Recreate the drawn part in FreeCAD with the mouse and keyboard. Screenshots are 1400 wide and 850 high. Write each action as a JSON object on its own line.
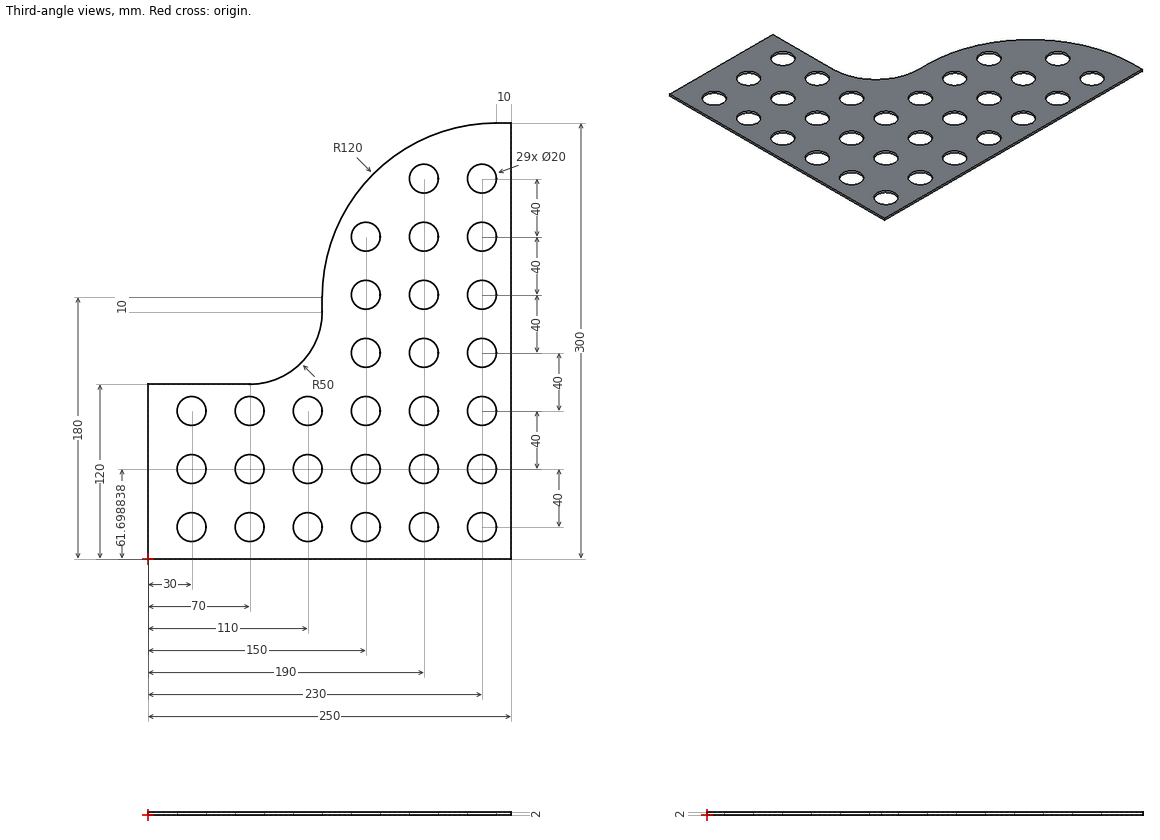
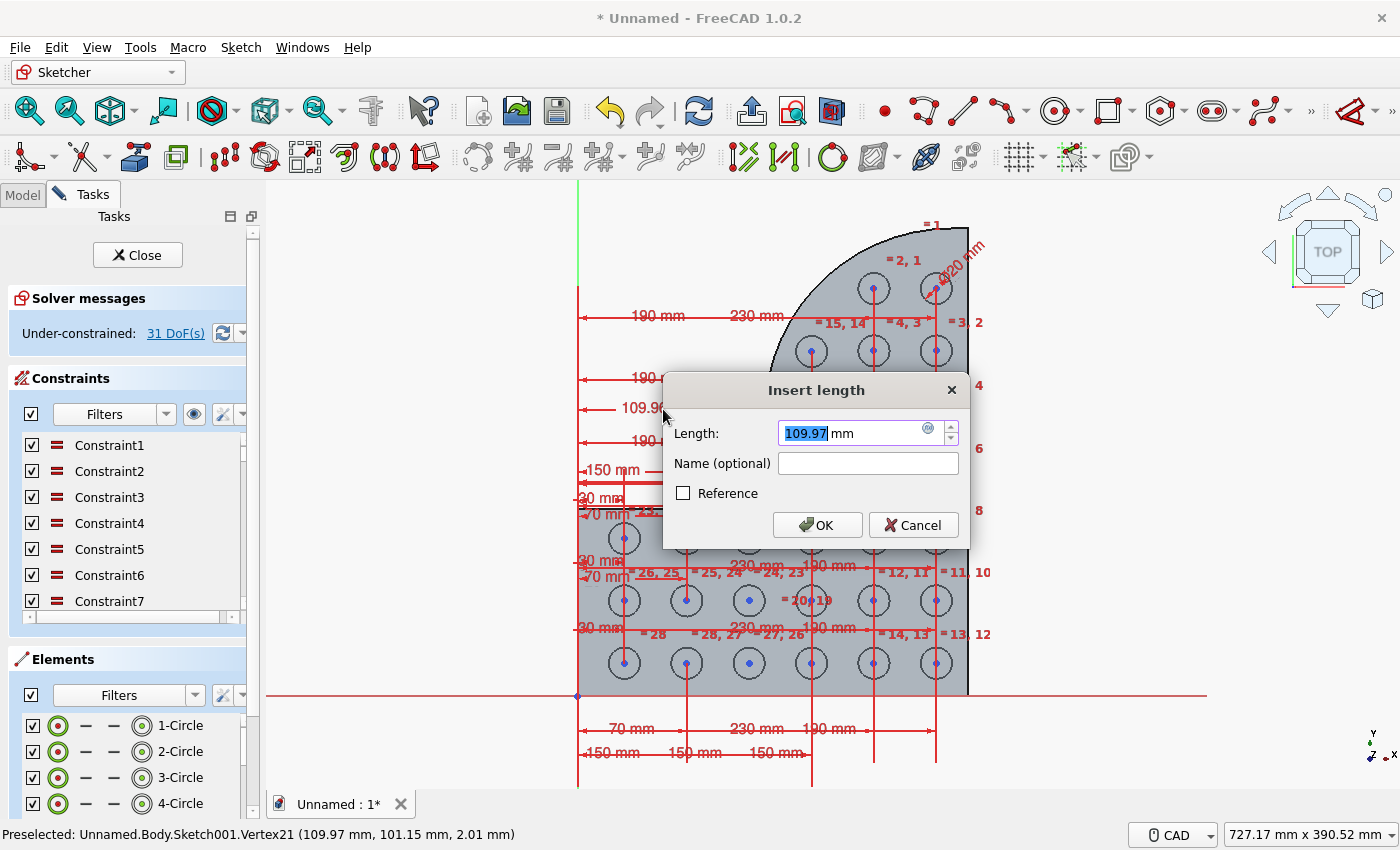
{"action": "type", "text": "110"}
{"action": "key", "text": "Return"}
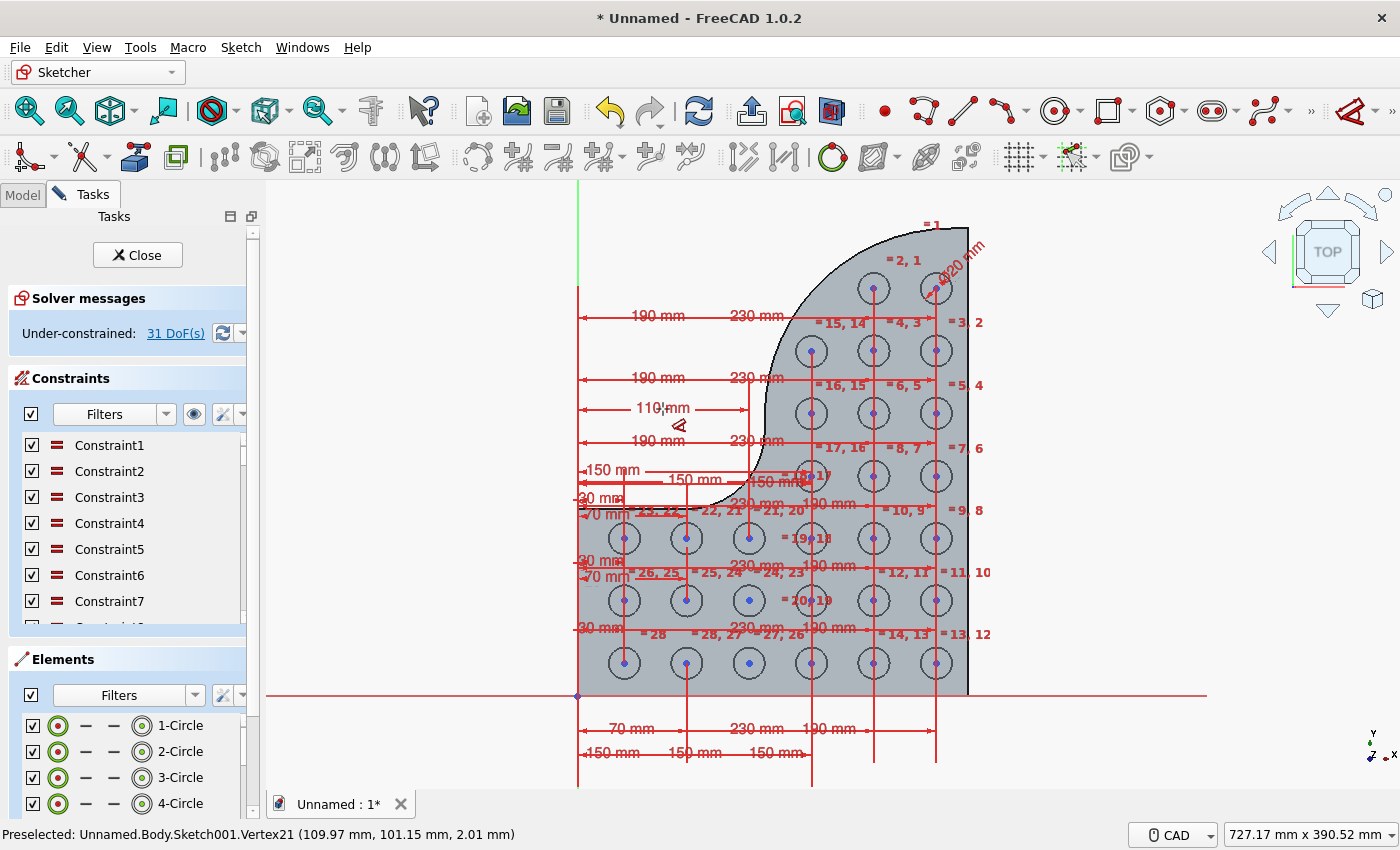
{"action": "left_click", "coordinate": [749, 601]}
{"action": "left_click", "coordinate": [703, 730]}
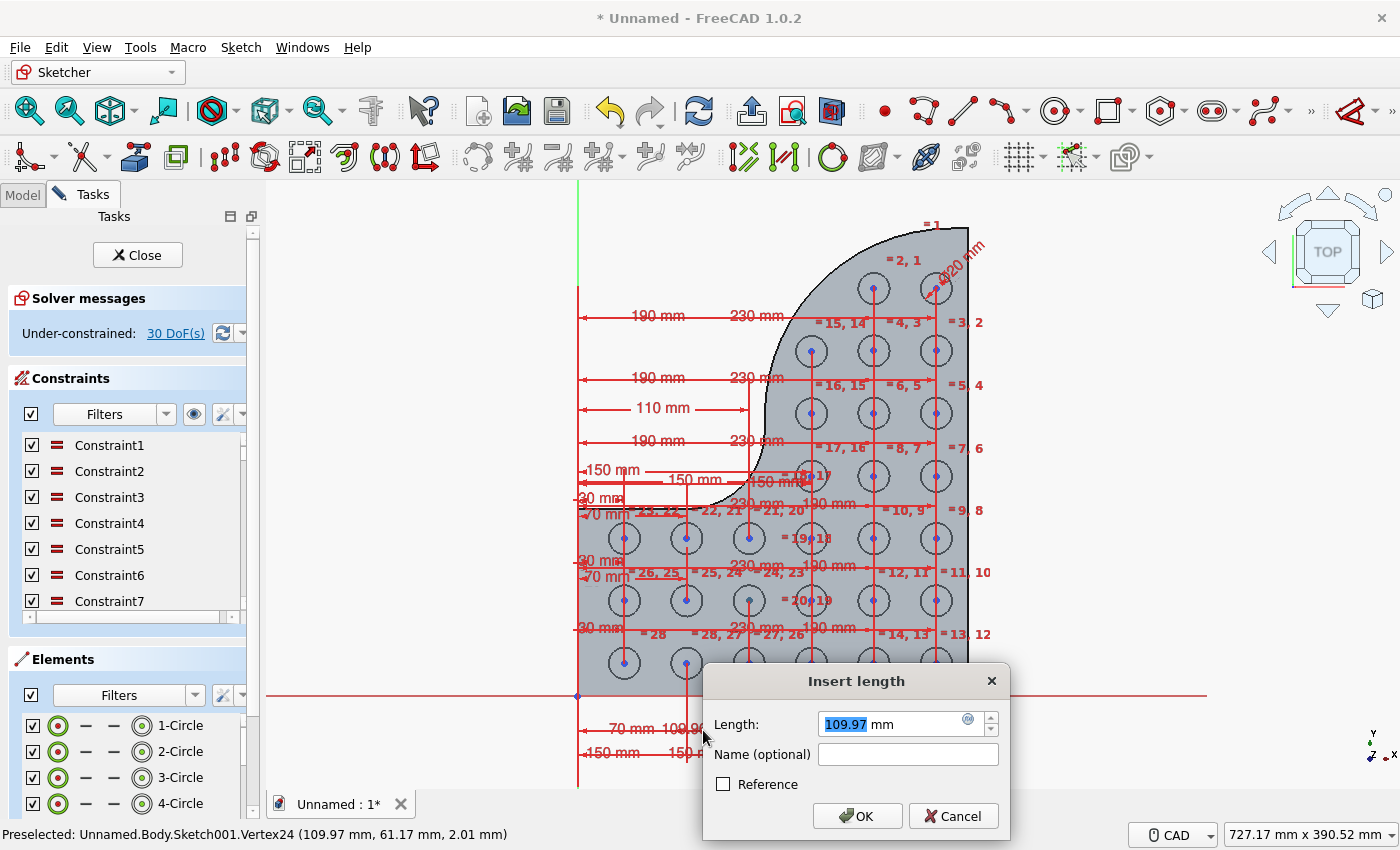
{"action": "type", "text": "110"}
{"action": "key", "text": "Return"}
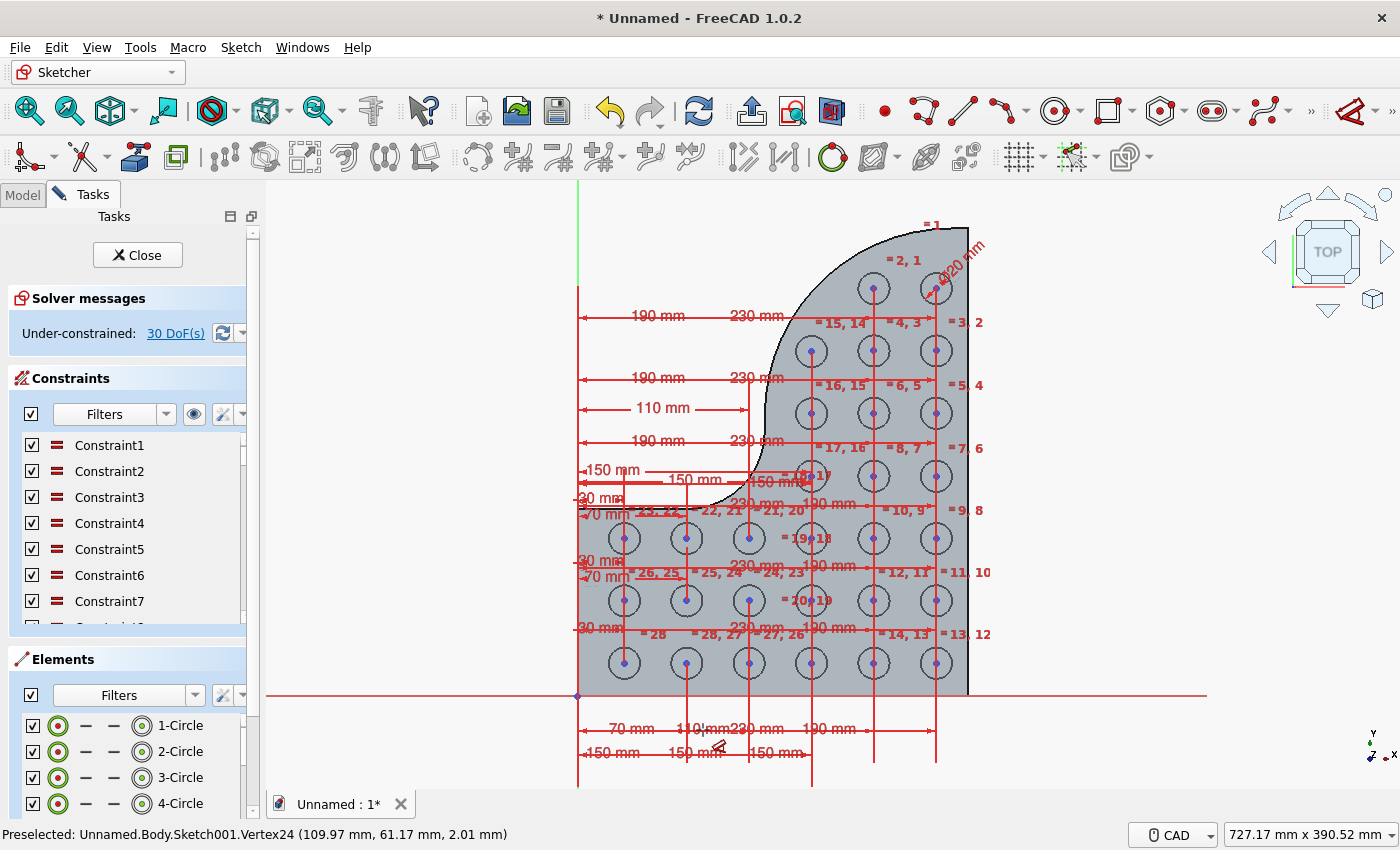
{"action": "left_click", "coordinate": [749, 663]}
{"action": "left_click", "coordinate": [663, 629]}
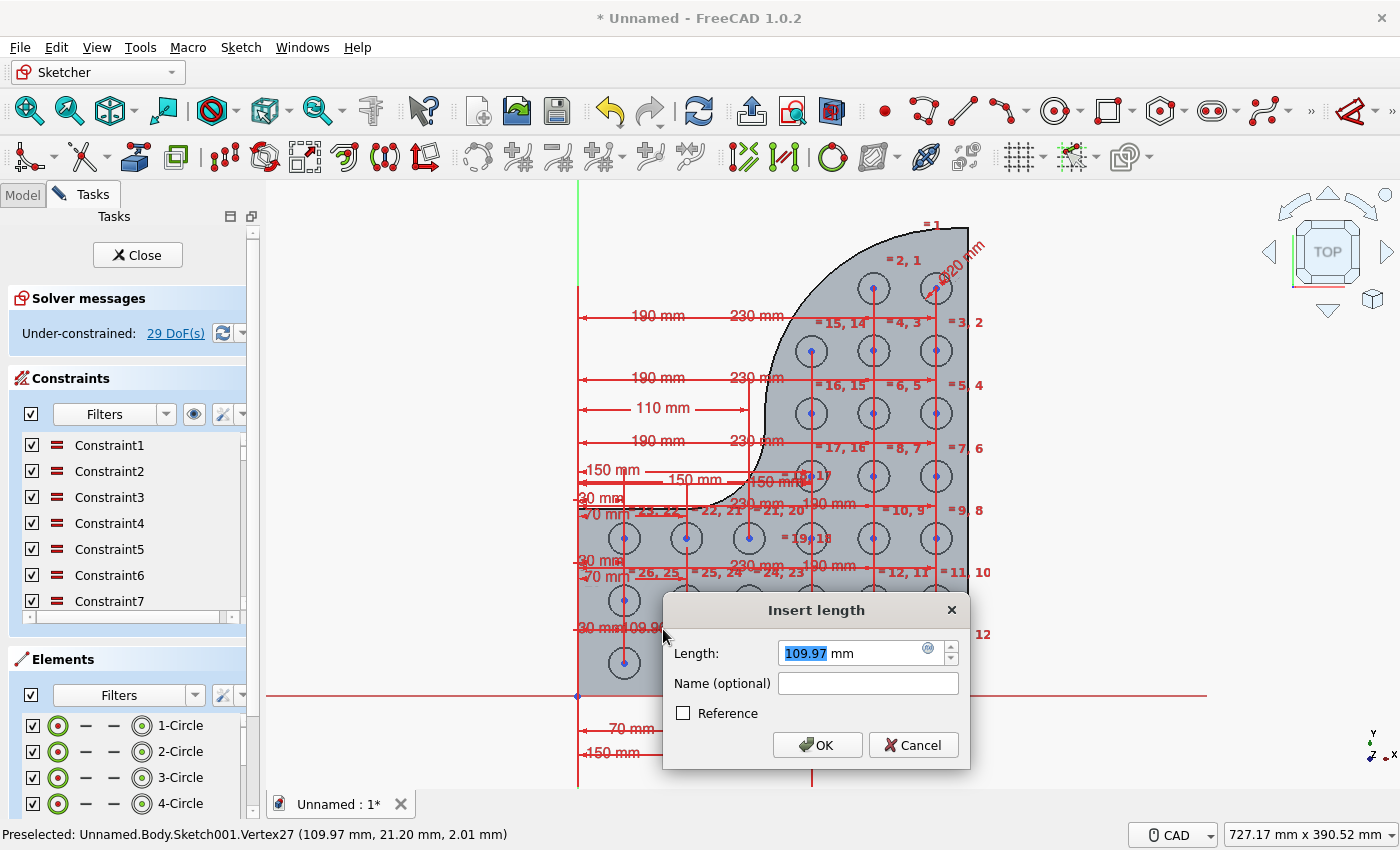
{"action": "type", "text": "110"}
{"action": "key", "text": "Return"}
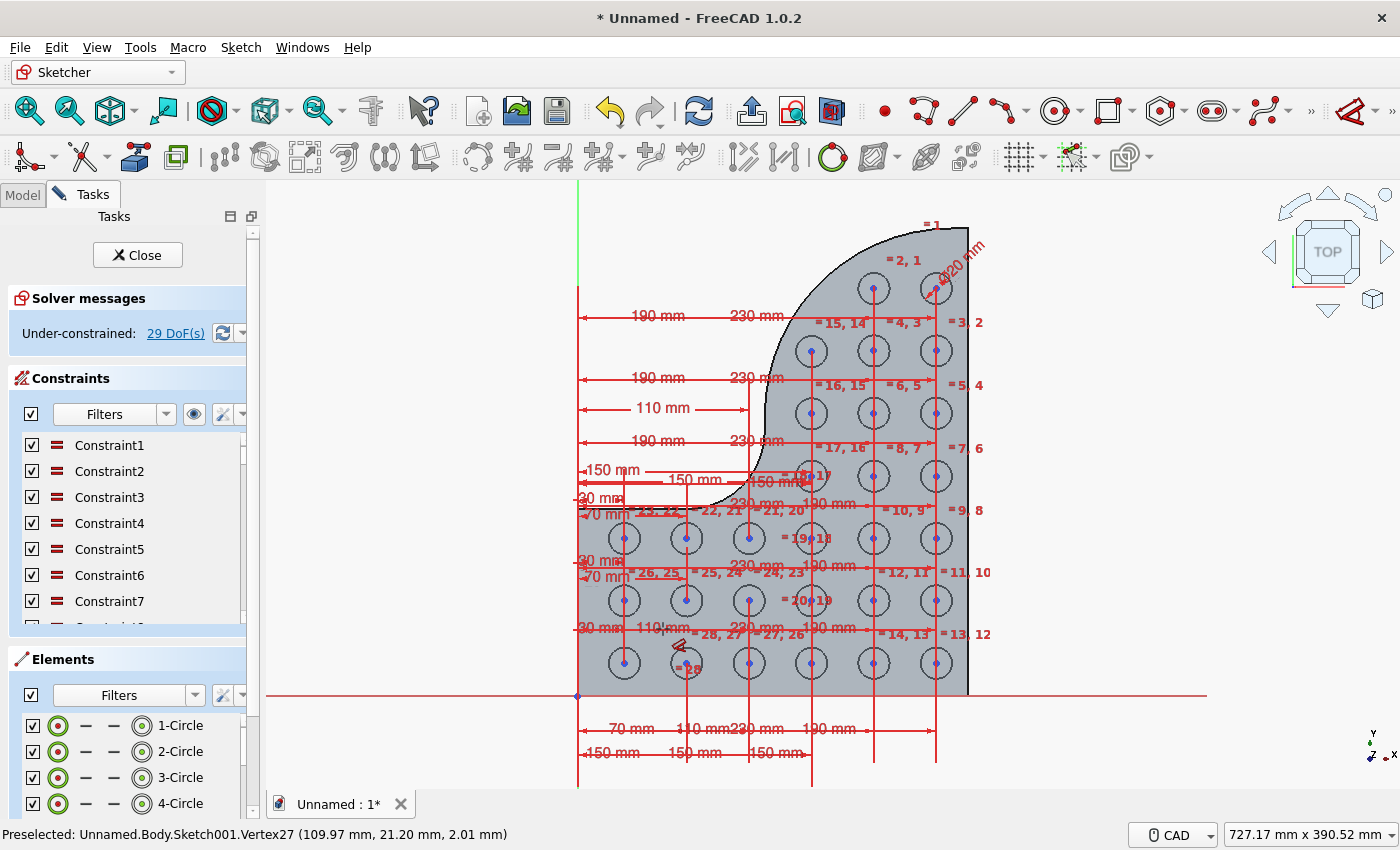
{"action": "left_click", "coordinate": [936, 289]}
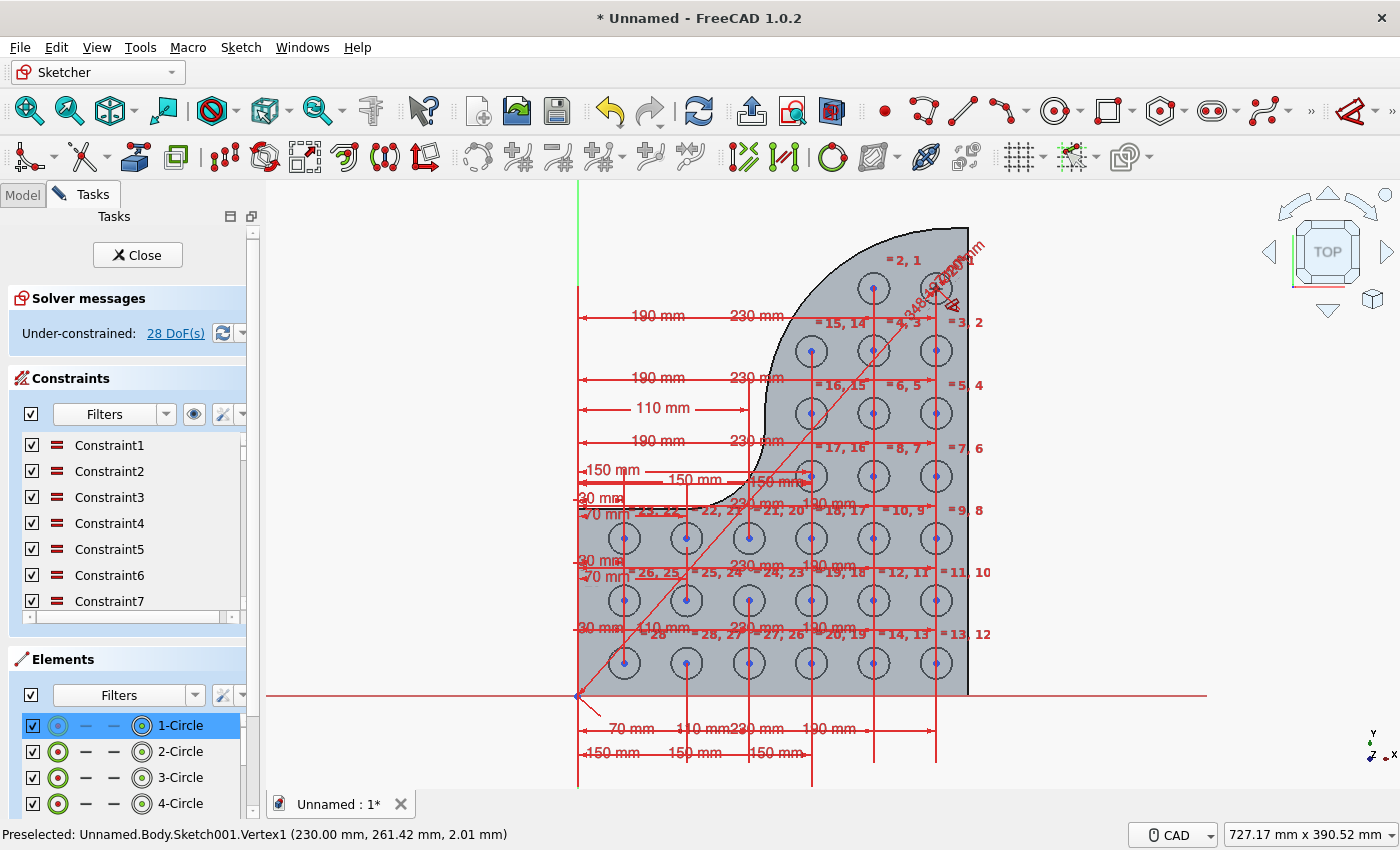
{"action": "left_click", "coordinate": [936, 351]}
{"action": "left_click", "coordinate": [970, 320]}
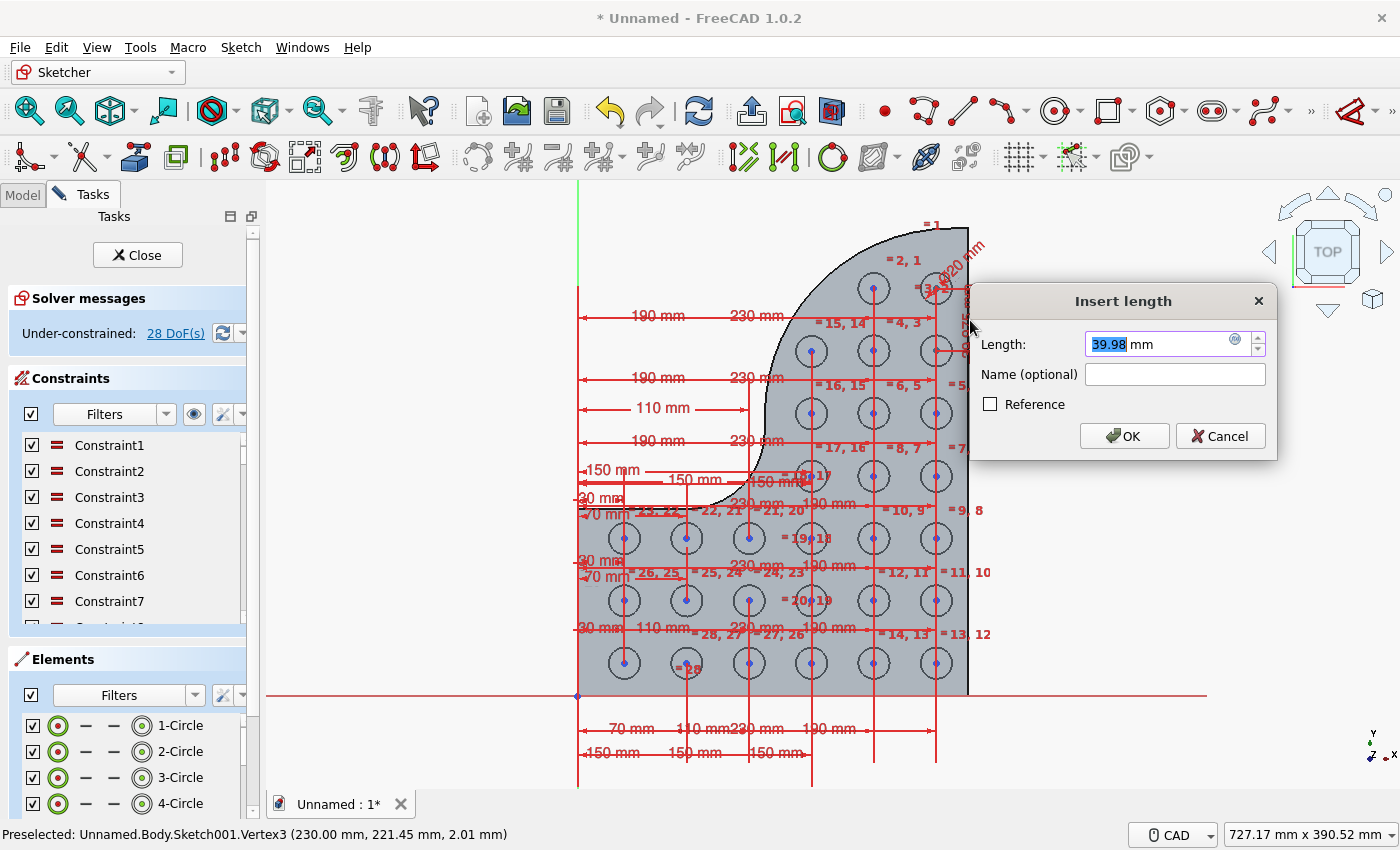
{"action": "type", "text": "40"}
{"action": "key", "text": "Return"}